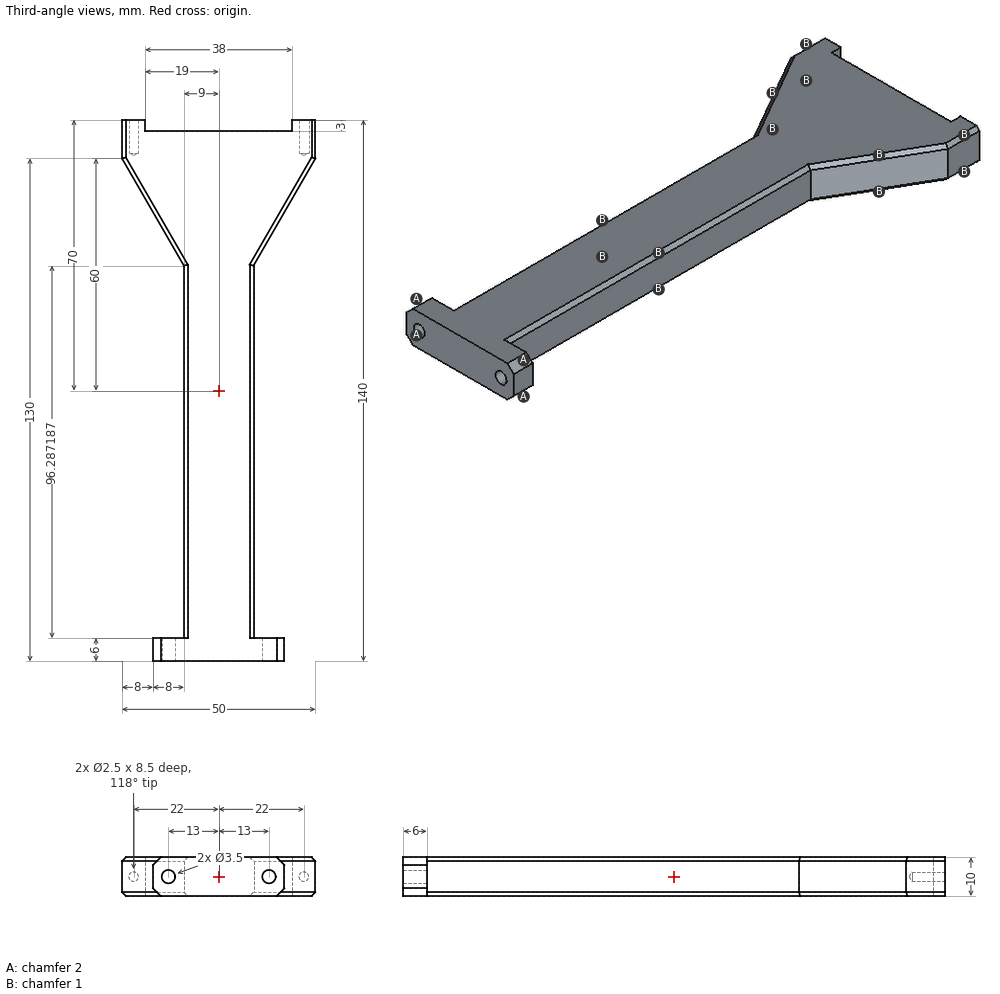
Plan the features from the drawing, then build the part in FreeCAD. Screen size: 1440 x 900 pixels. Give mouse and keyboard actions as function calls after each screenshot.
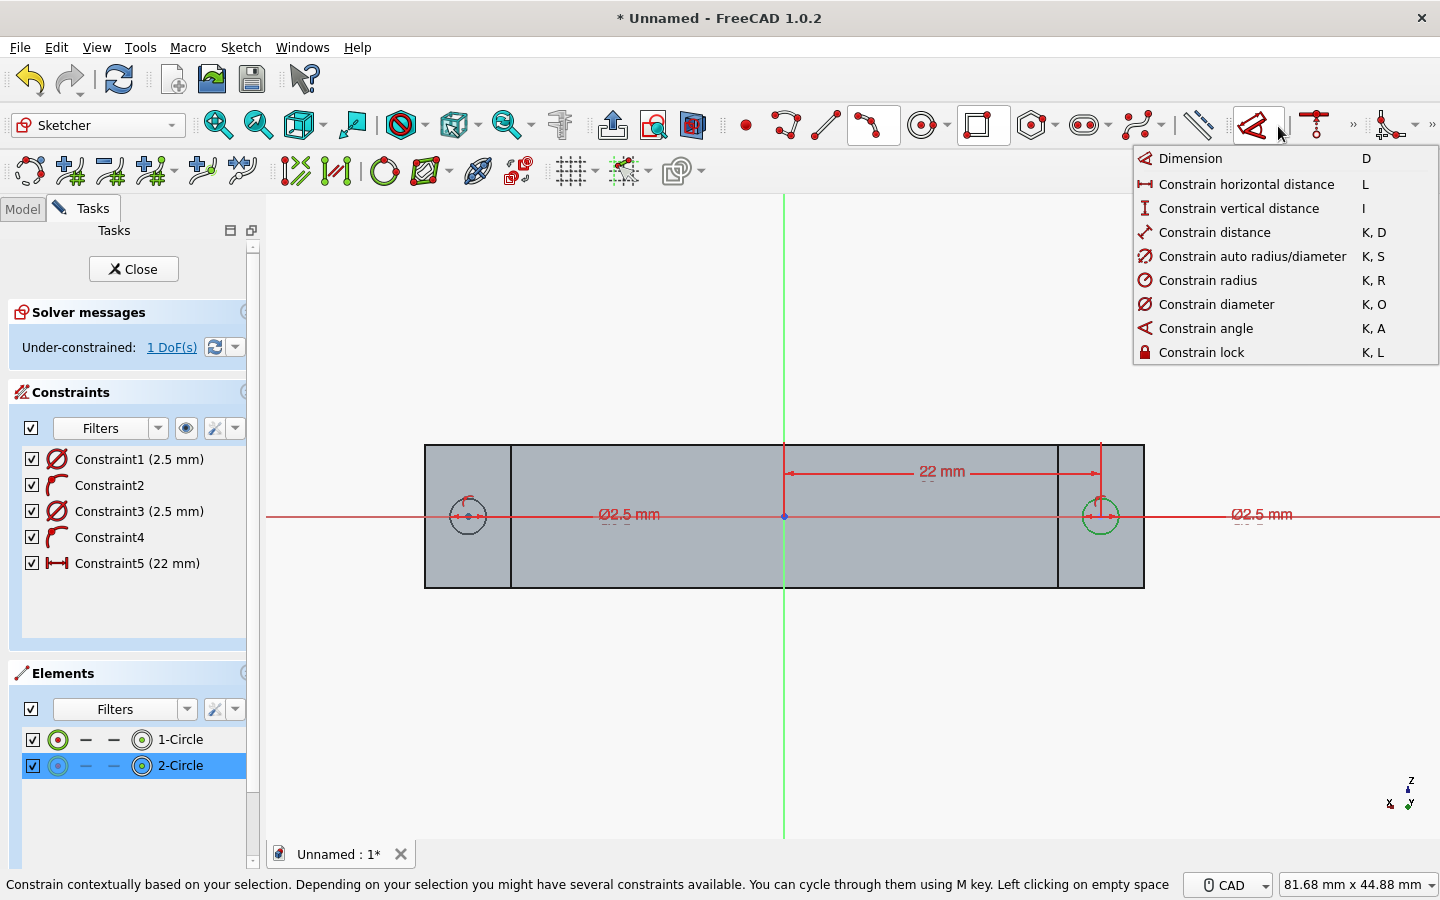
click(1286, 184)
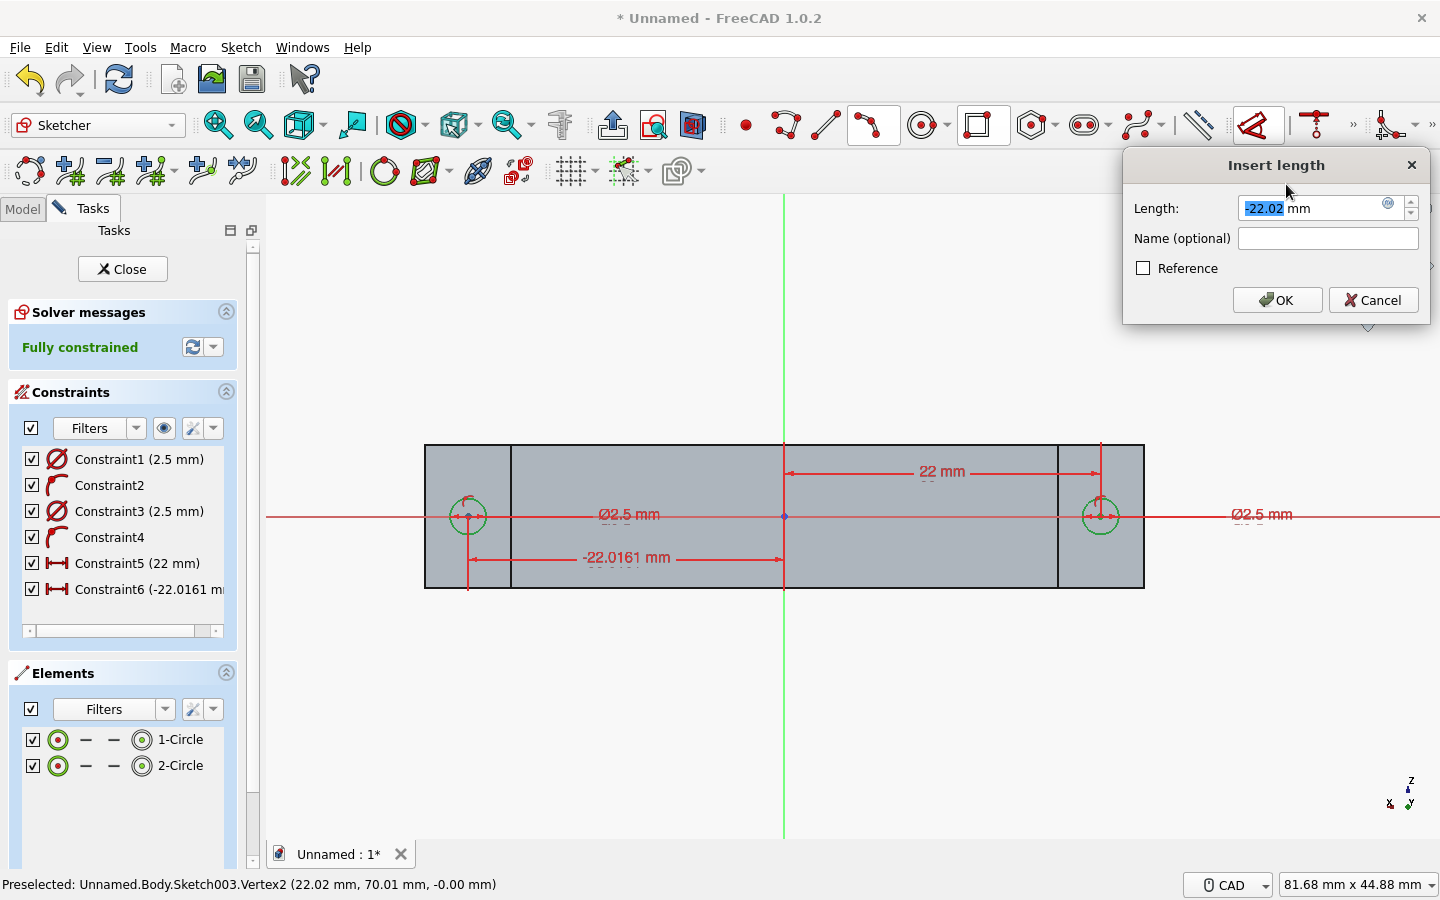
text(-22)
key(Return)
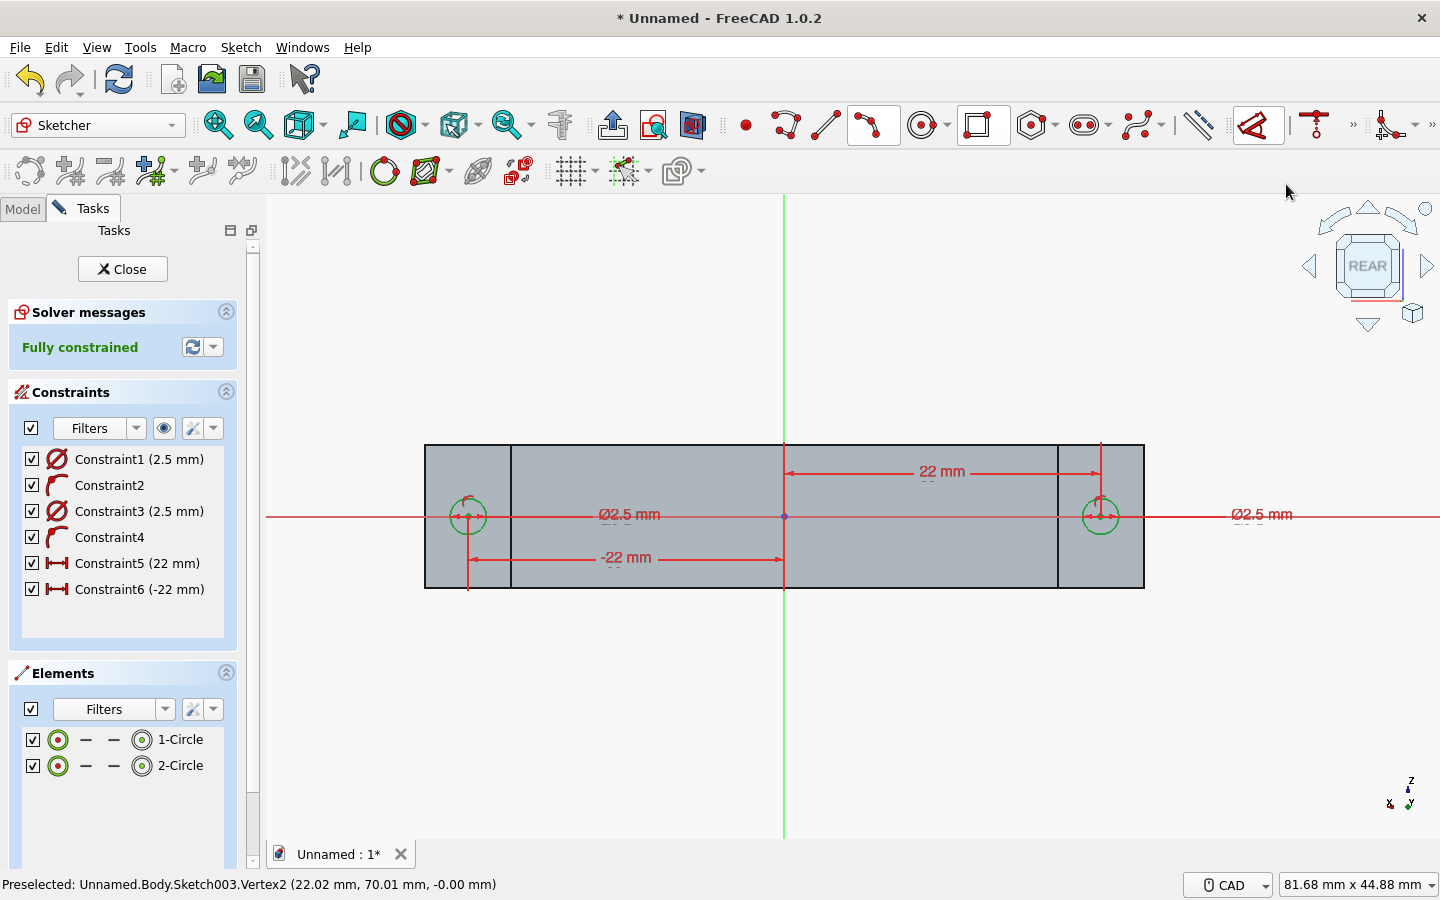
click(123, 269)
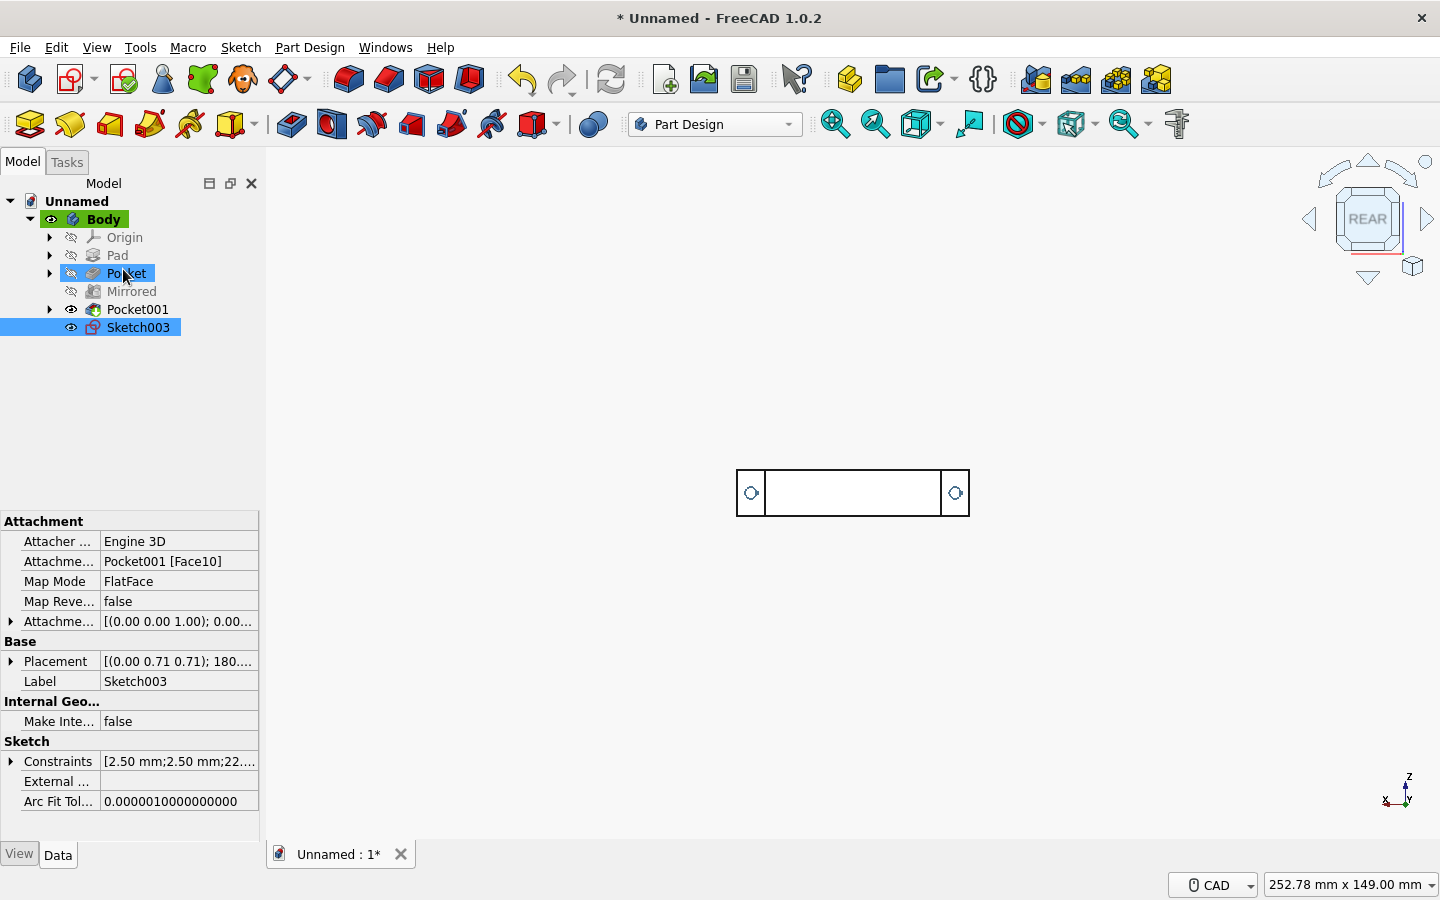
click(332, 124)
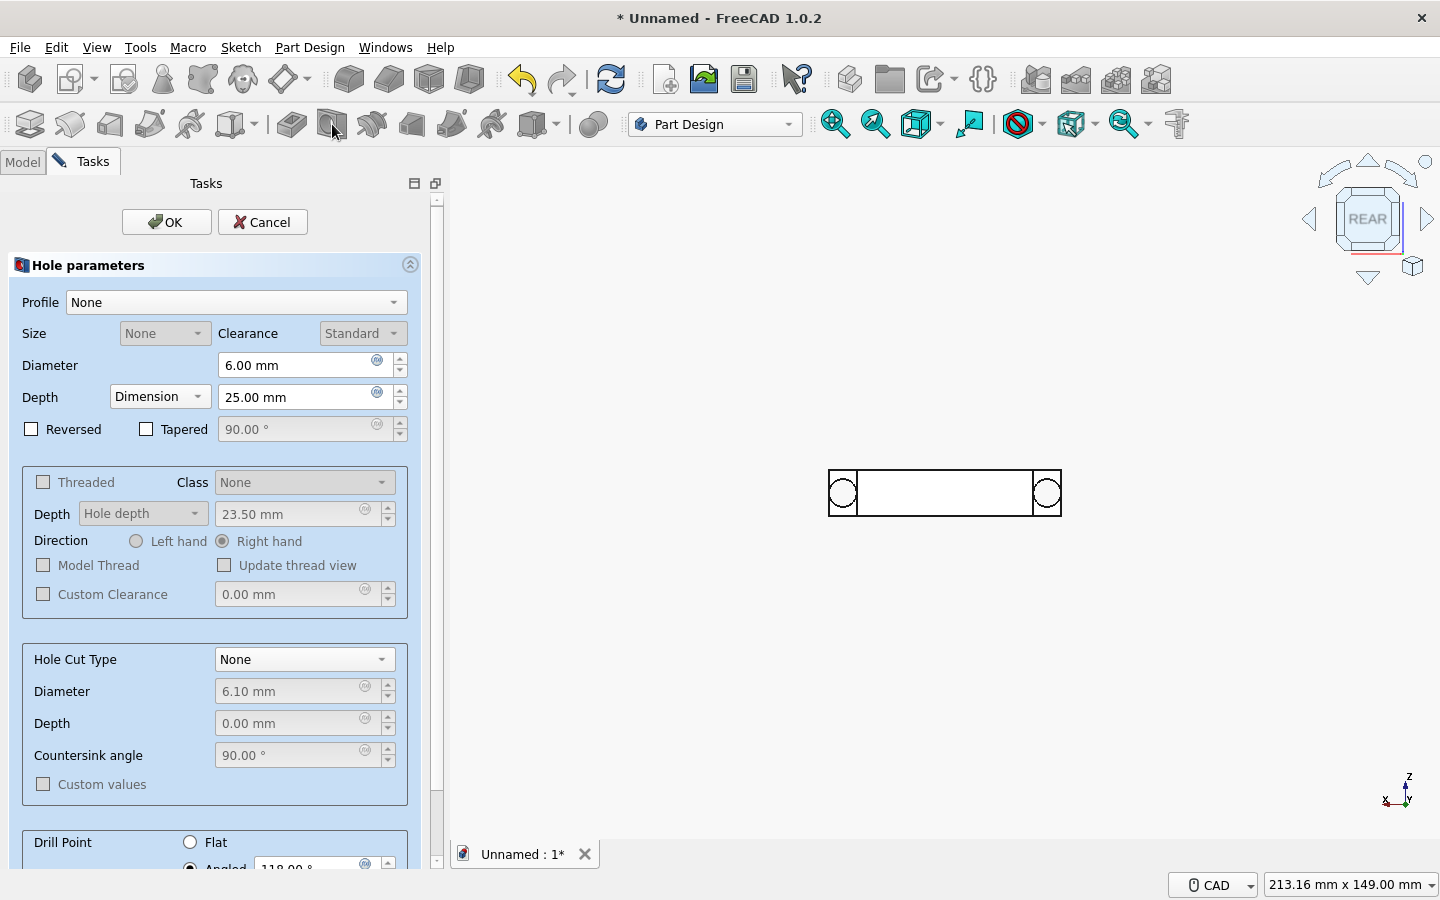
triple_click(305, 365)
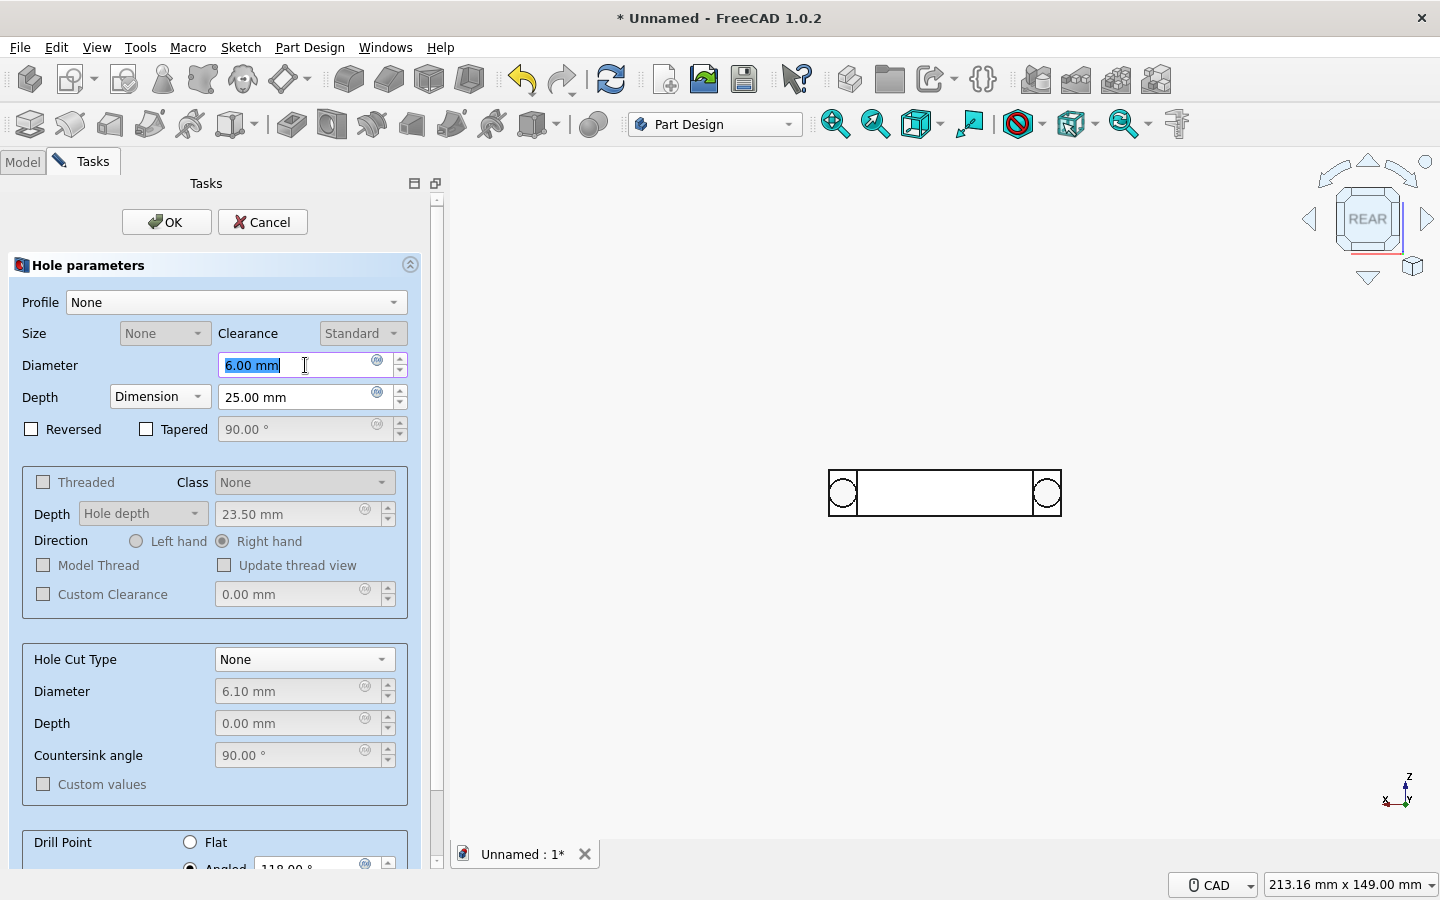
text(2.5)
key(Tab)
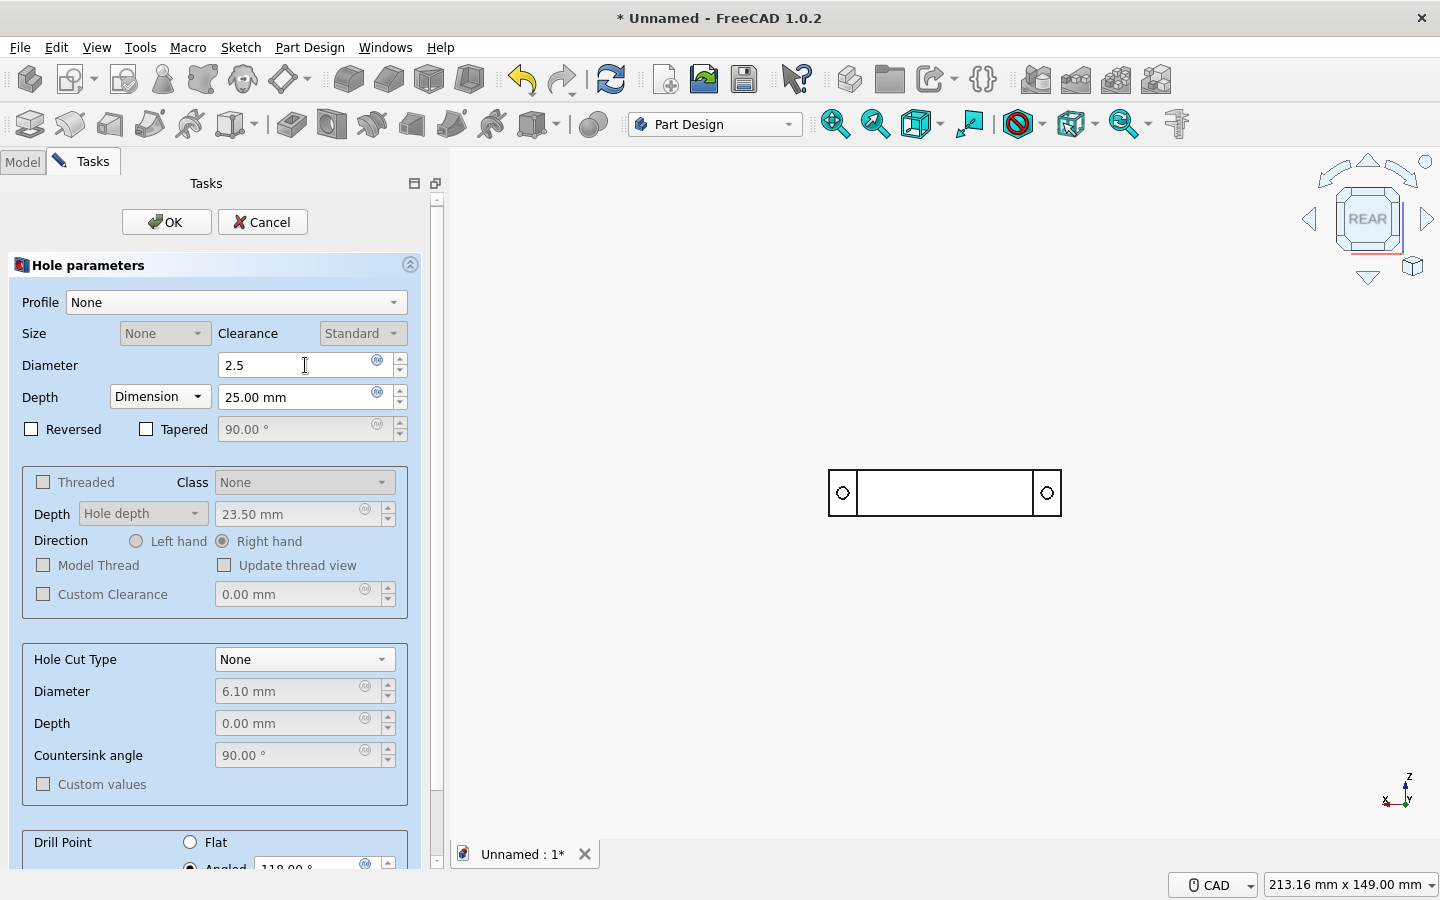
triple_click(305, 397)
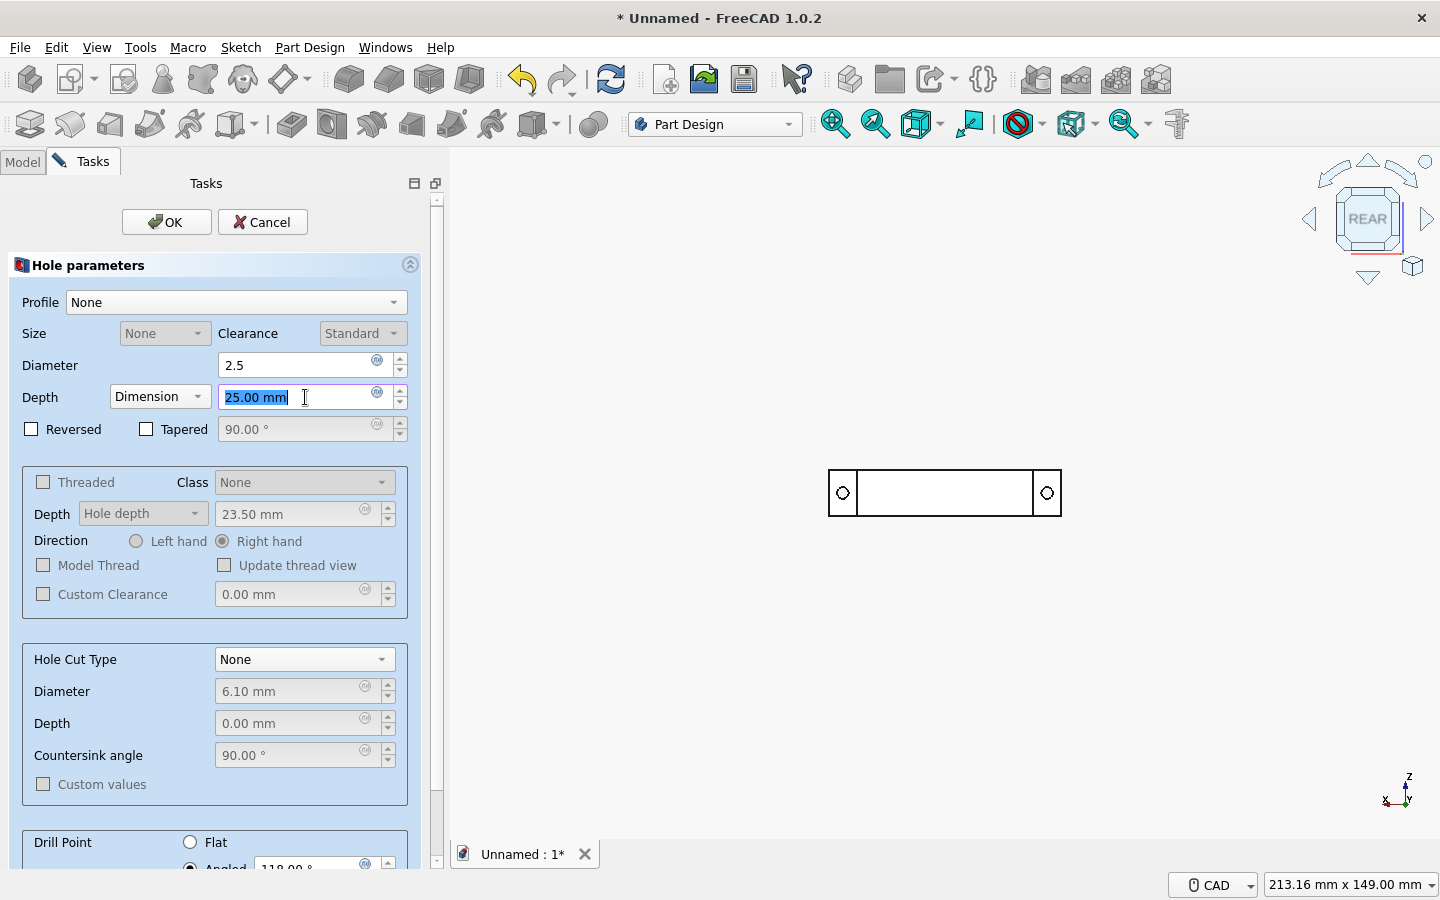
text(8.5)
key(Tab)